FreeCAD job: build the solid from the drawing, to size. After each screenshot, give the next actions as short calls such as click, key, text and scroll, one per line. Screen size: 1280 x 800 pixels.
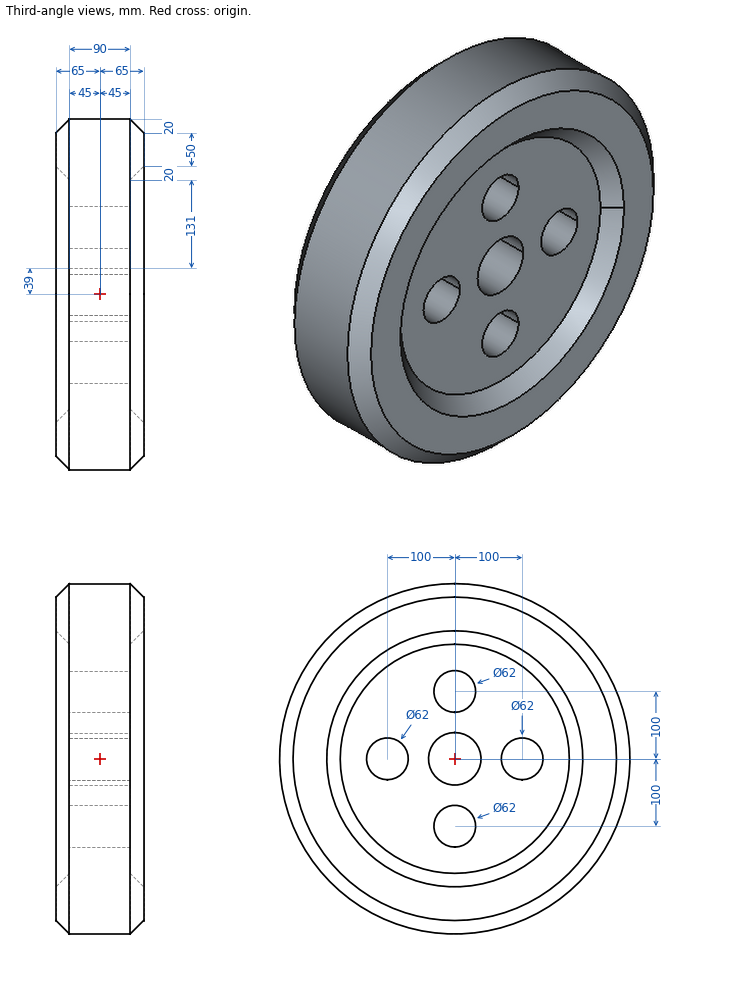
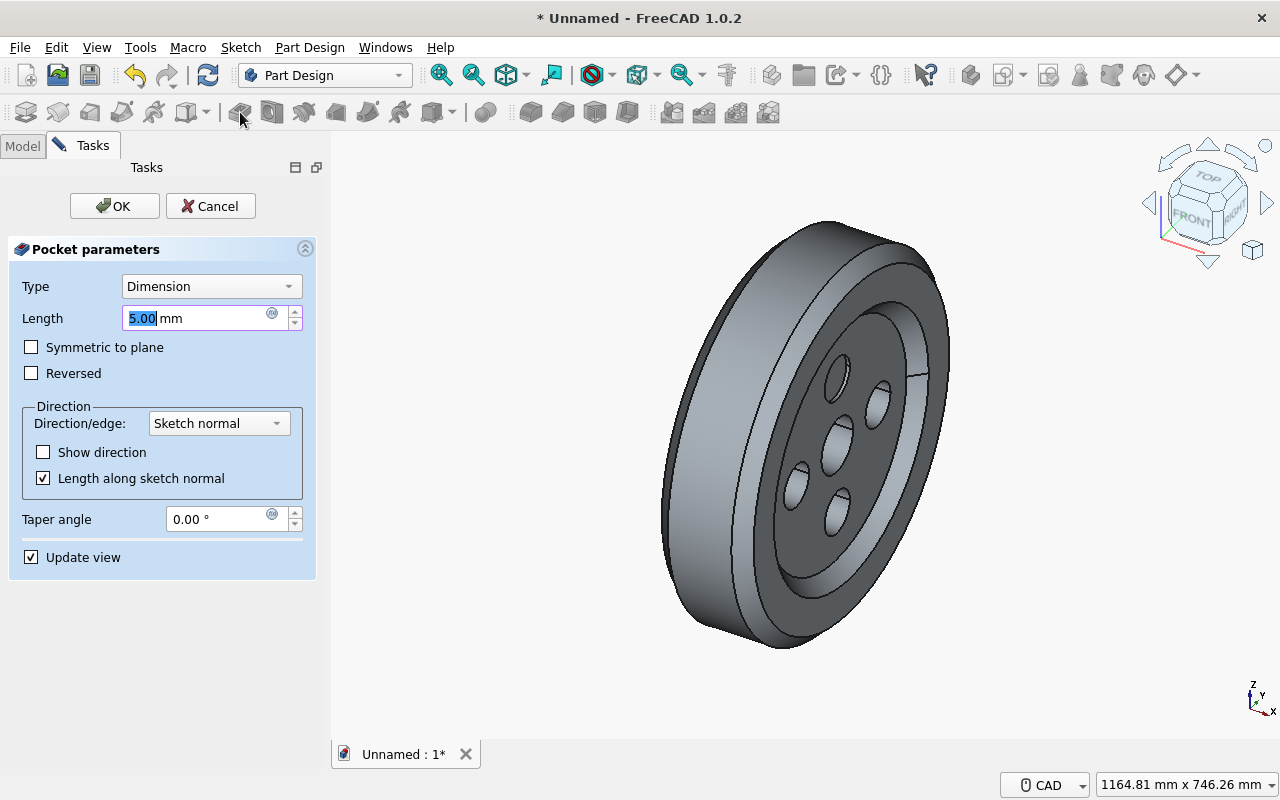
click(212, 286)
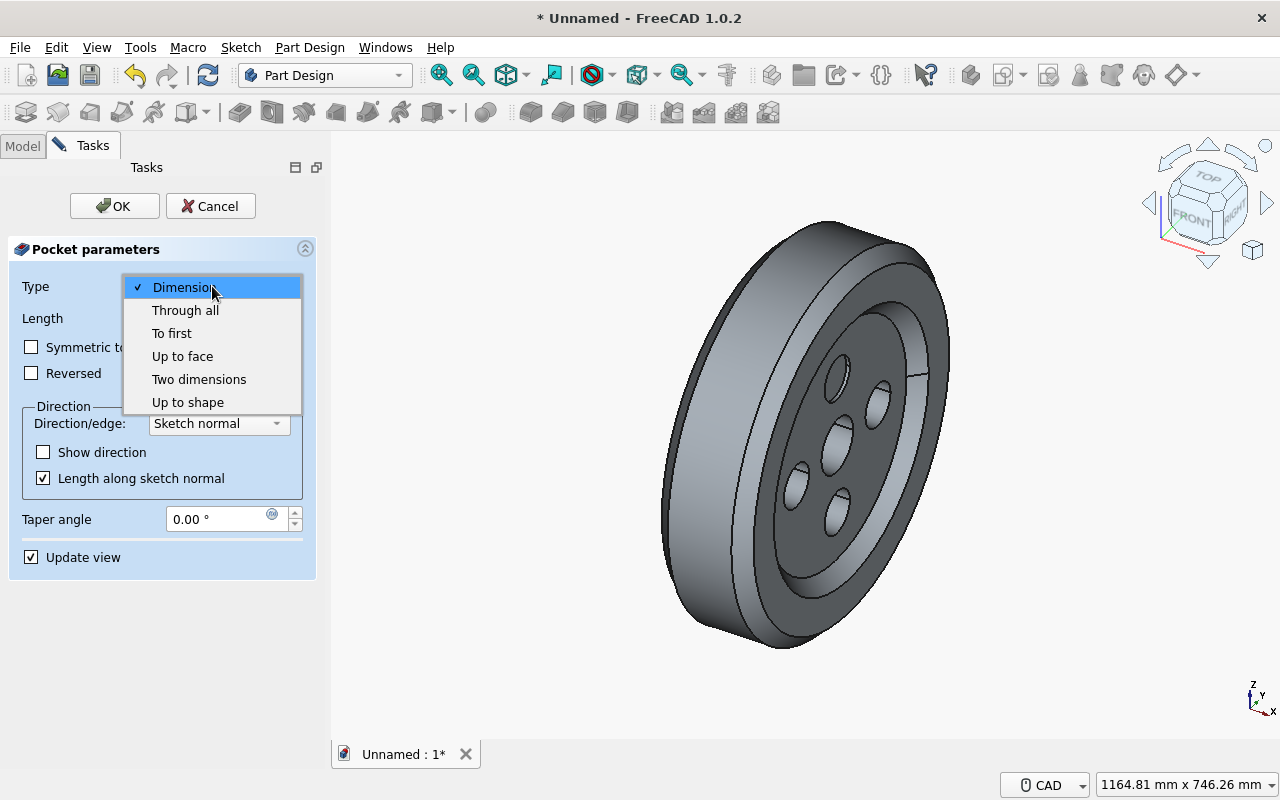
click(212, 334)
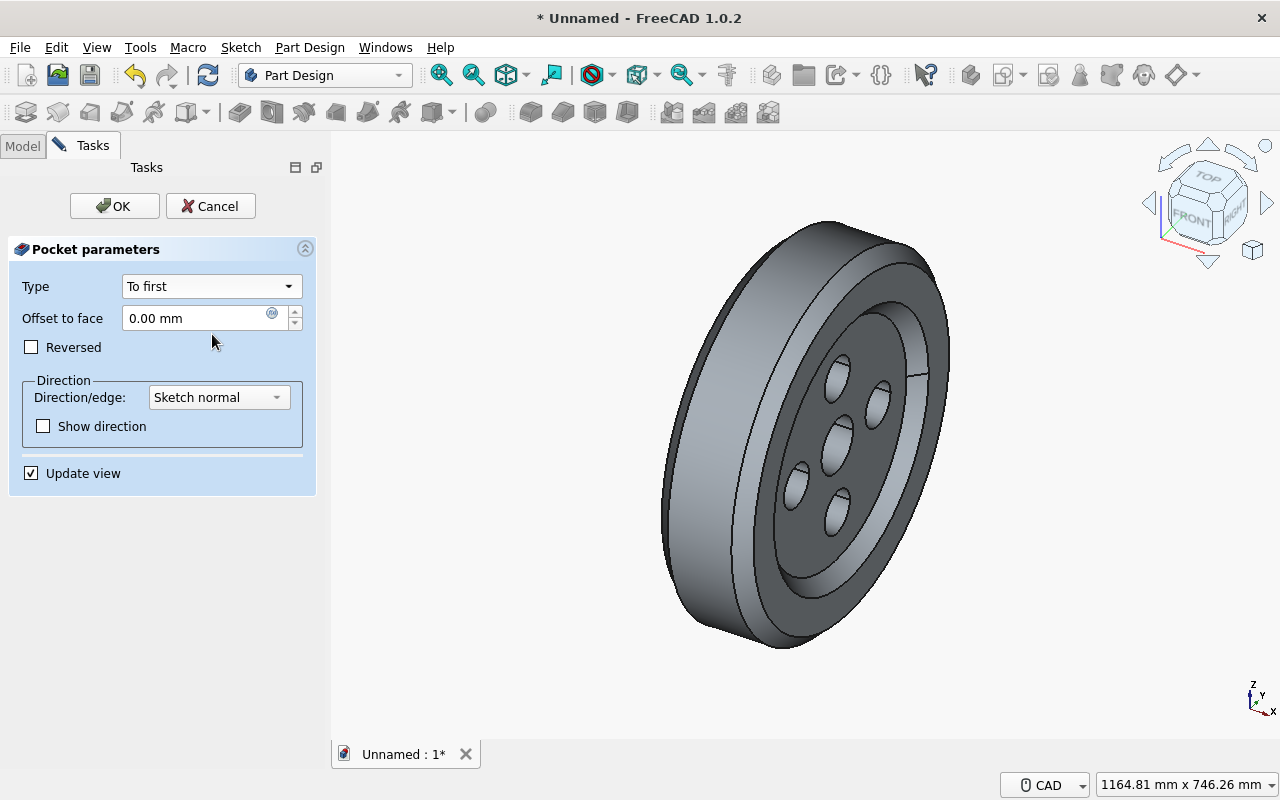
click(115, 206)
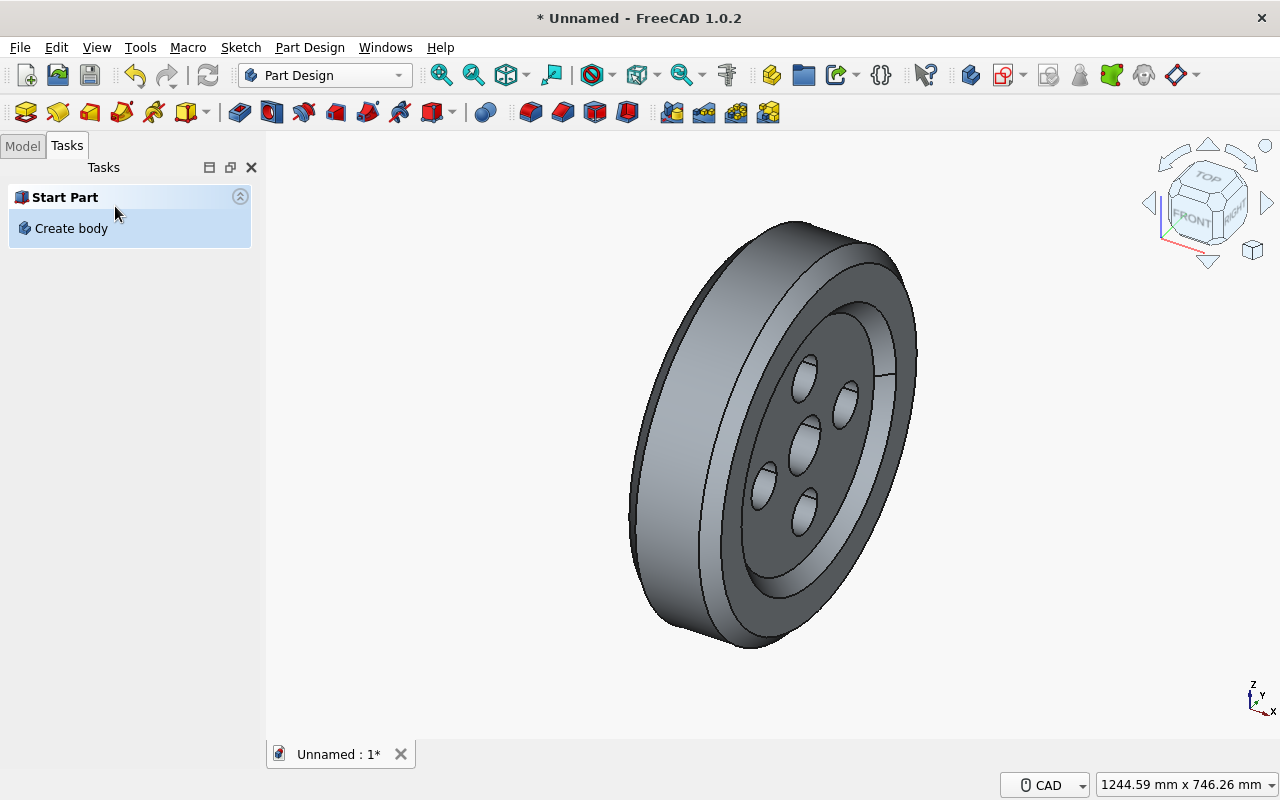
key(0)